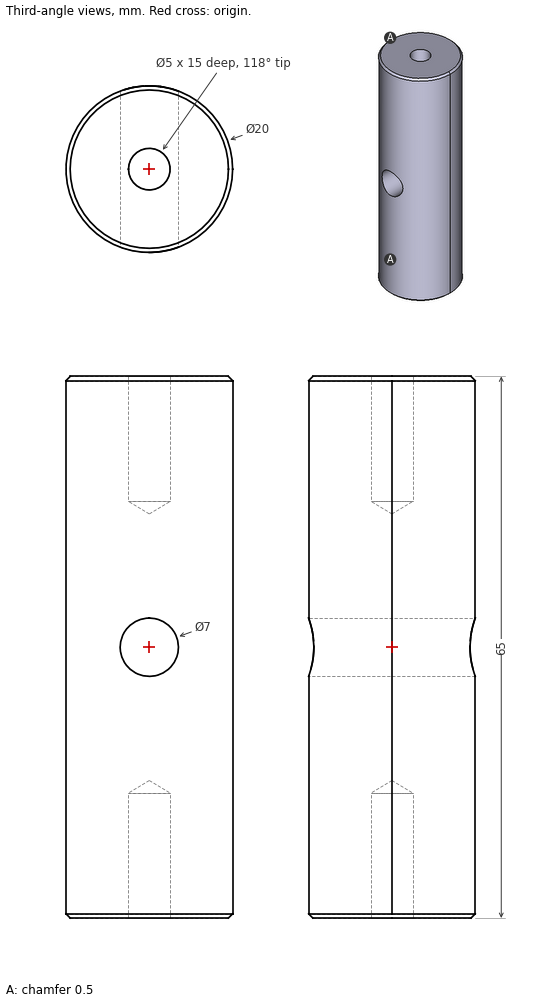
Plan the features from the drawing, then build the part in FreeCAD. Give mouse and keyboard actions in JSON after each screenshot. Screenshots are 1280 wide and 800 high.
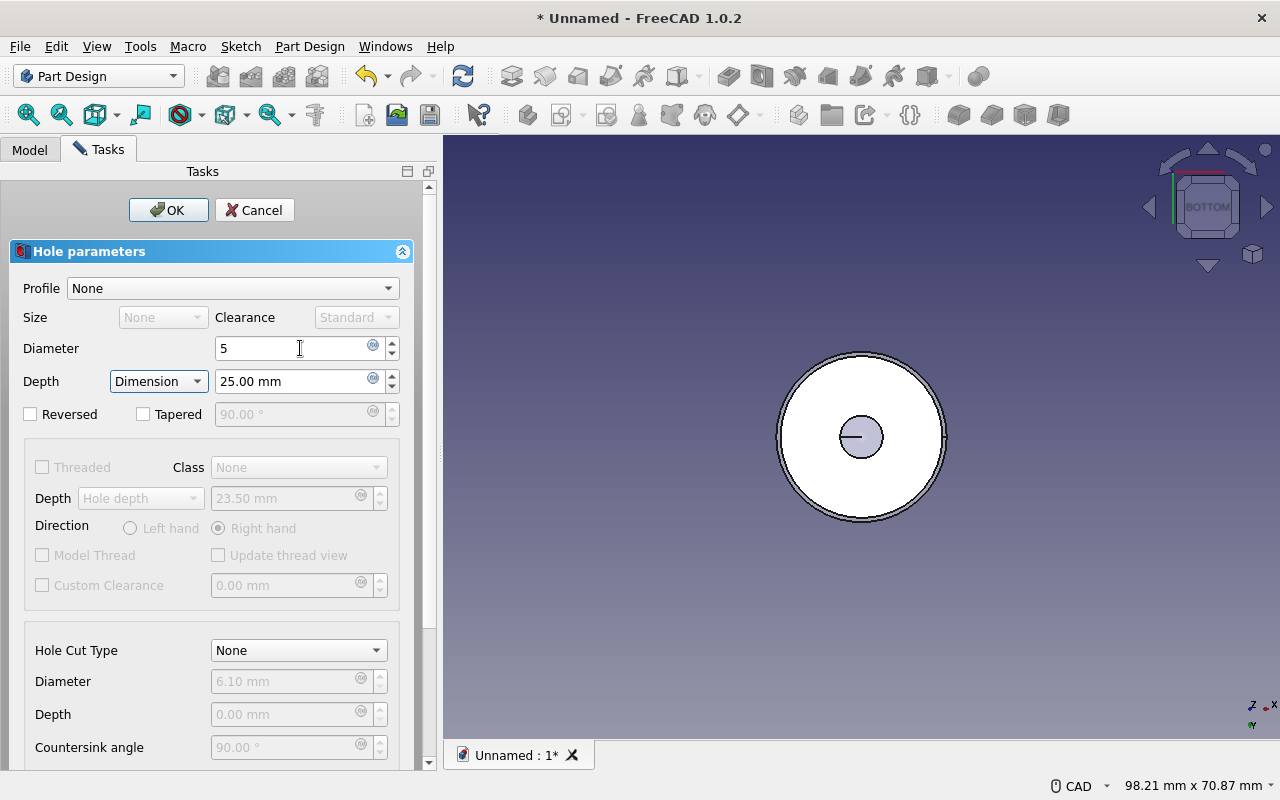
{"action": "triple_click", "coordinate": [300, 382]}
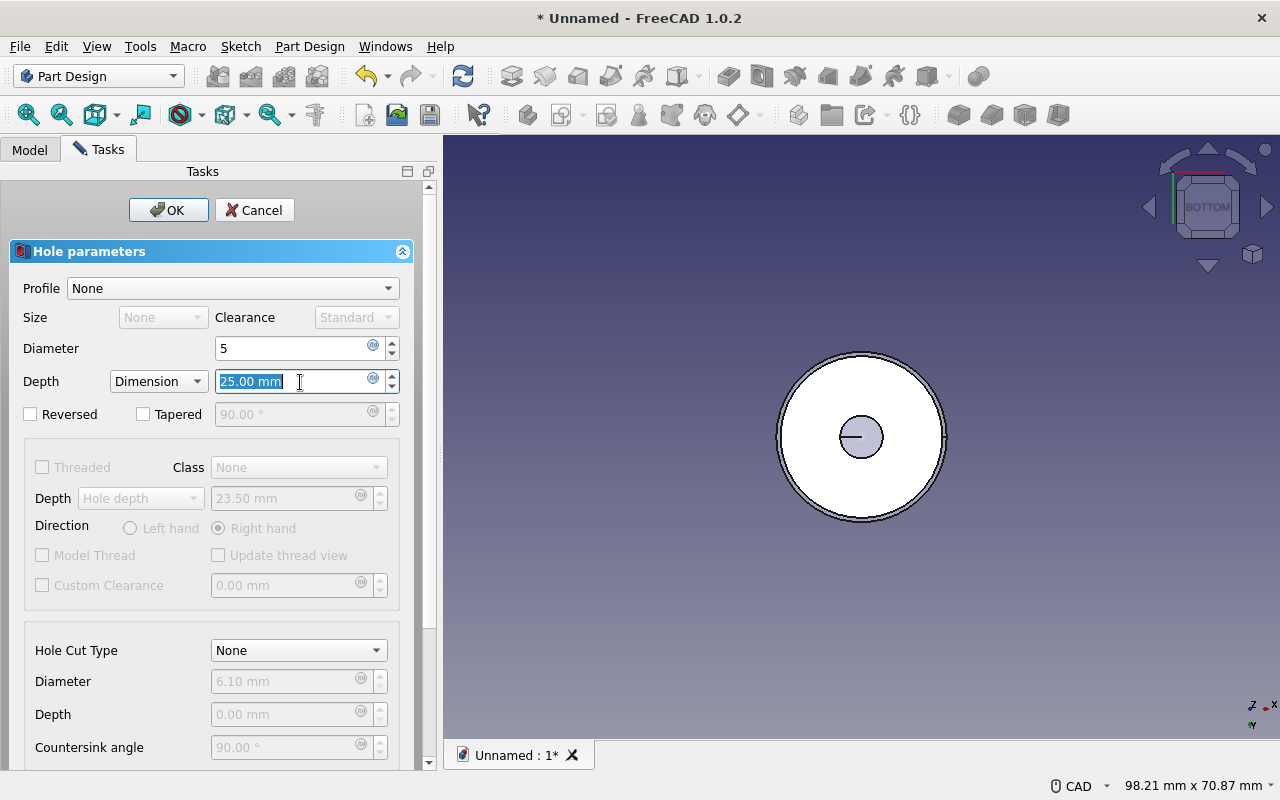
{"action": "type", "text": "15"}
{"action": "key", "text": "Tab"}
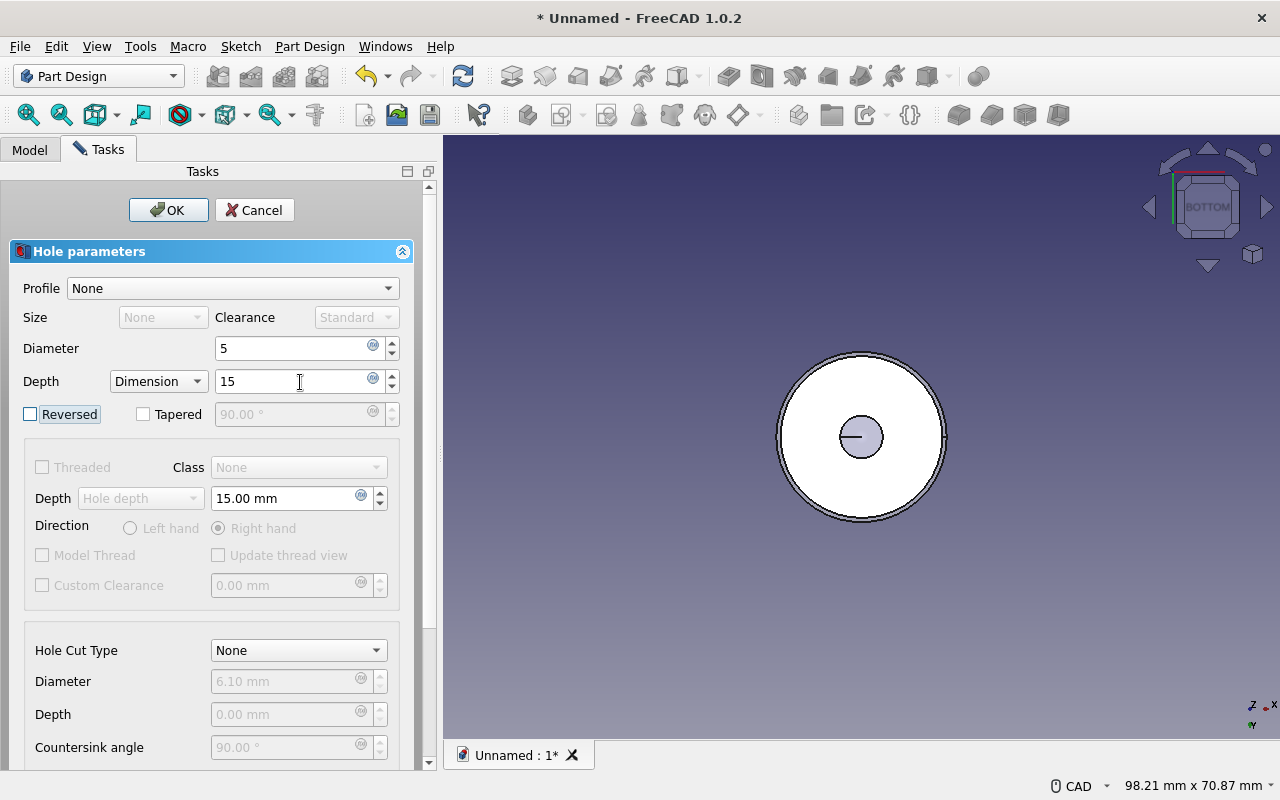
{"action": "left_click", "coordinate": [169, 210]}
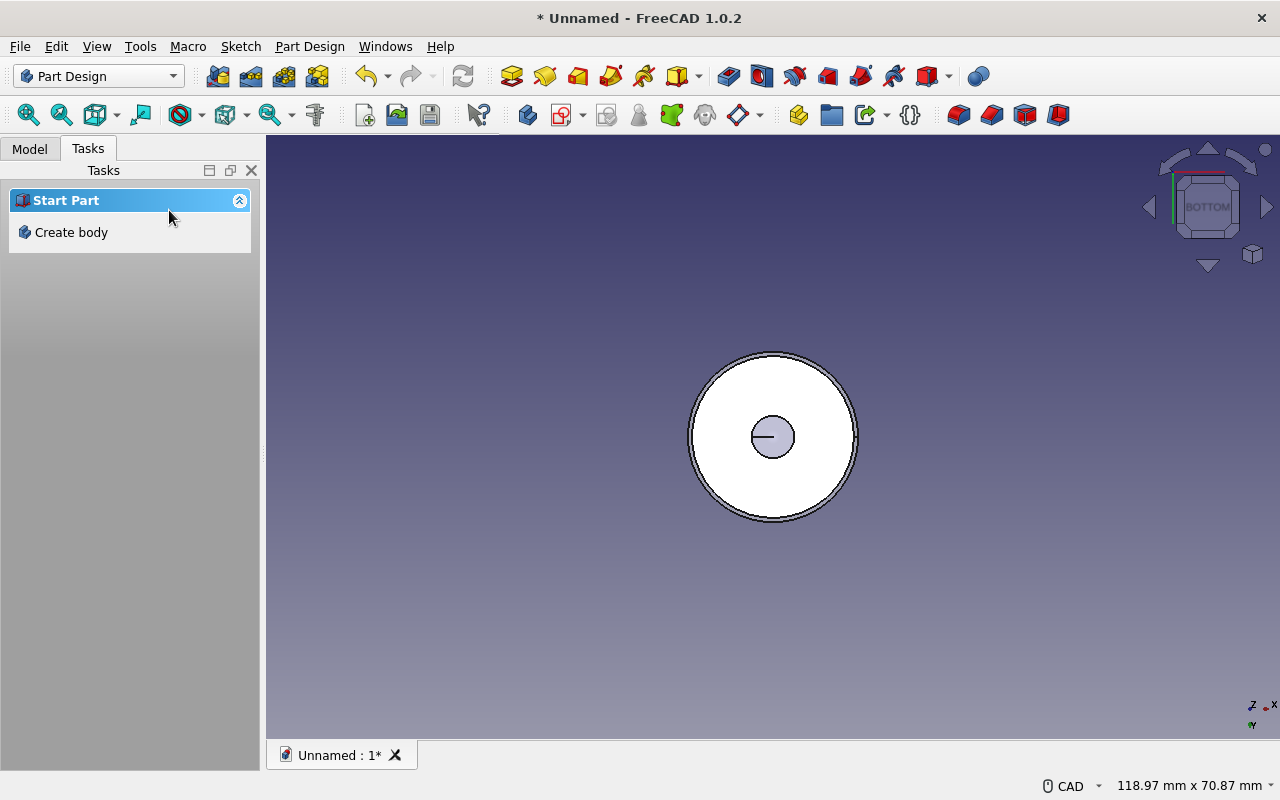
{"action": "left_click", "coordinate": [29, 116]}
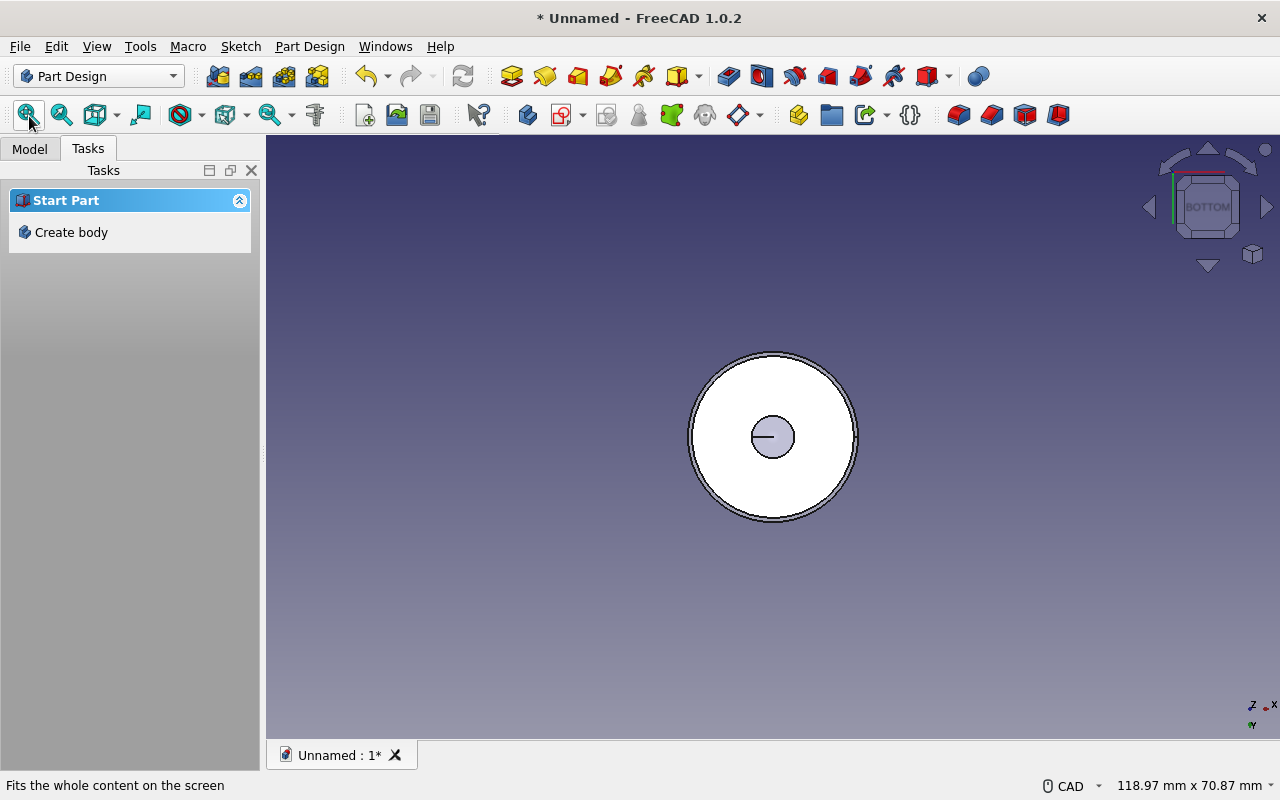
{"action": "left_click", "coordinate": [560, 116]}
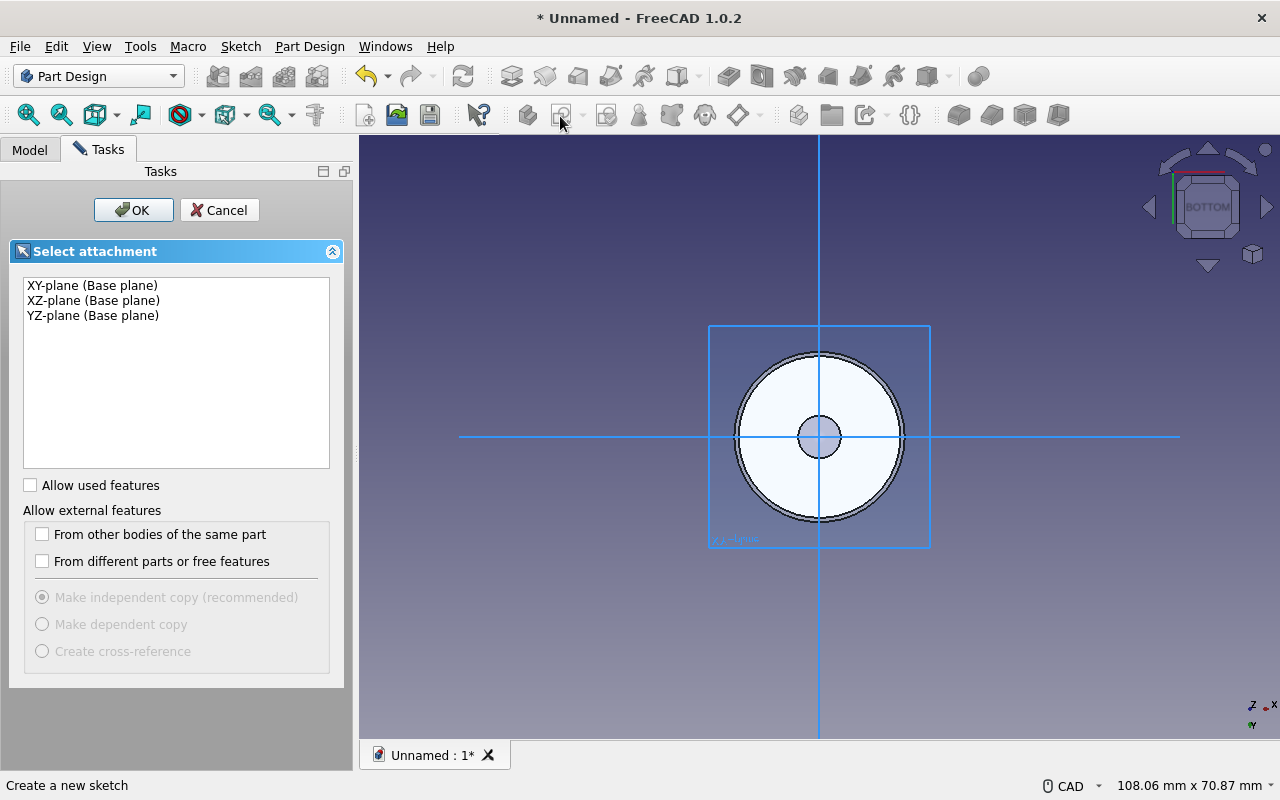
{"action": "left_click", "coordinate": [84, 300]}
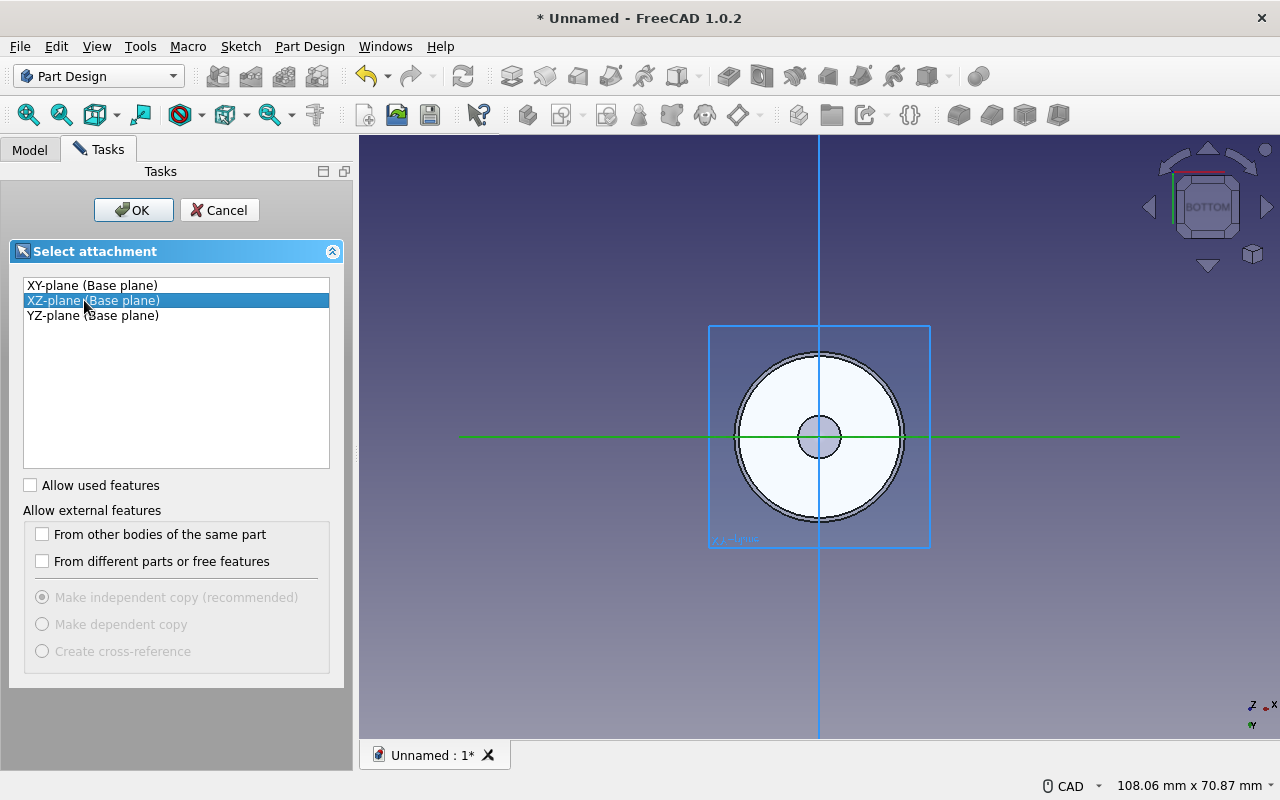
{"action": "left_click", "coordinate": [134, 210]}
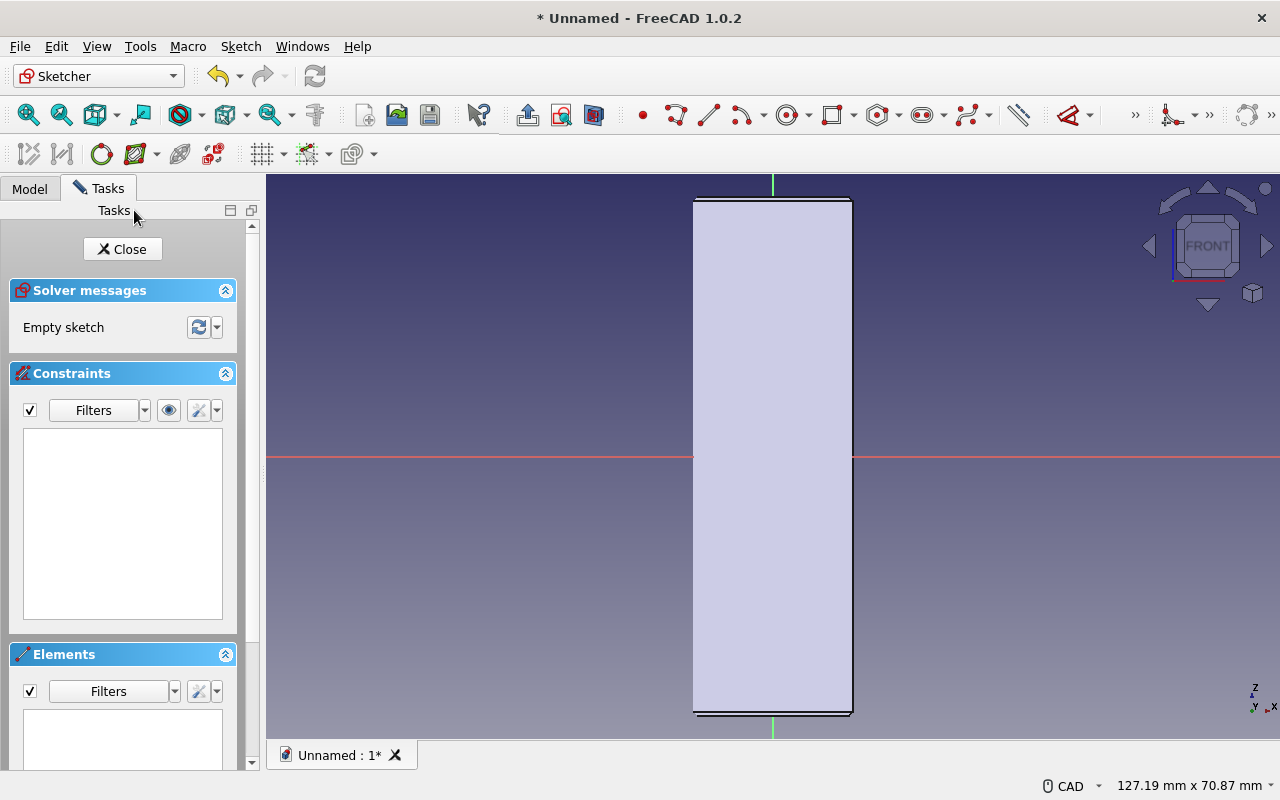
{"action": "left_click", "coordinate": [594, 116]}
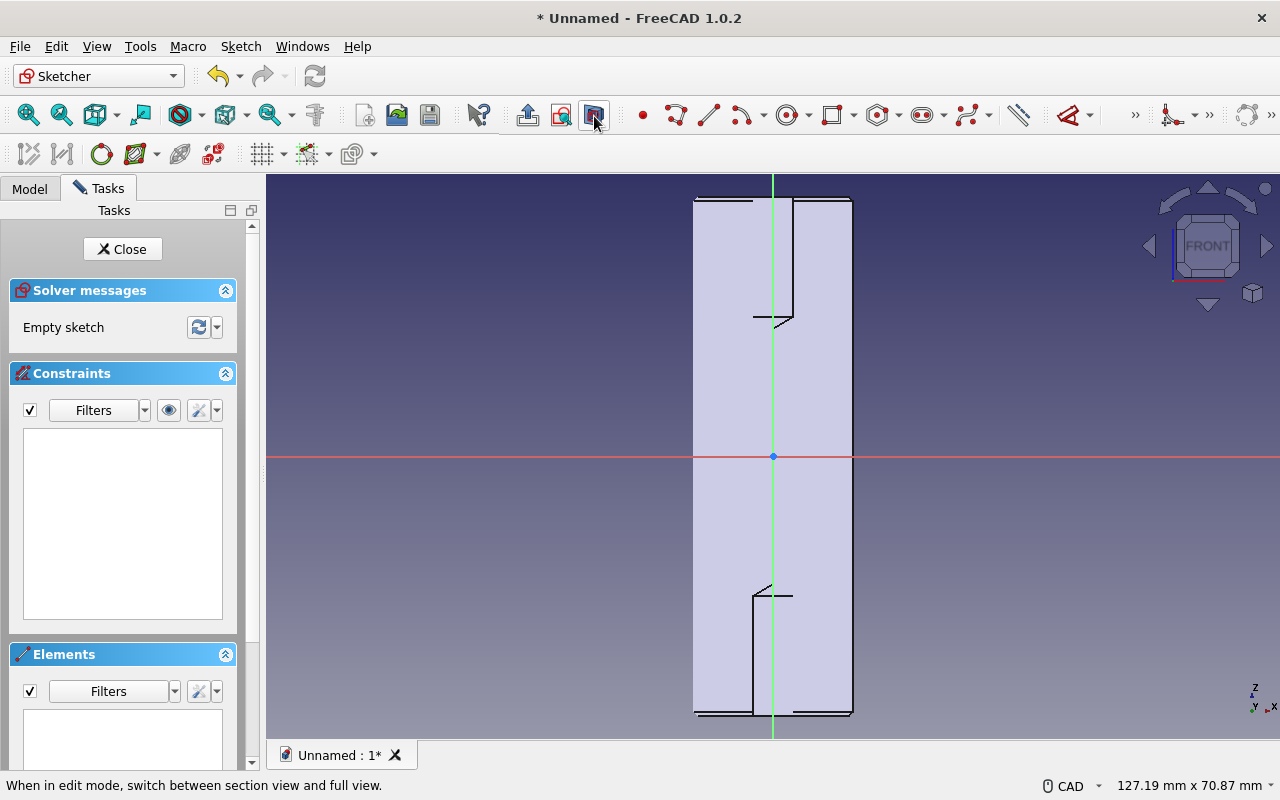
{"action": "scroll", "coordinate": [787, 456], "scroll_direction": "up", "scroll_amount": 9}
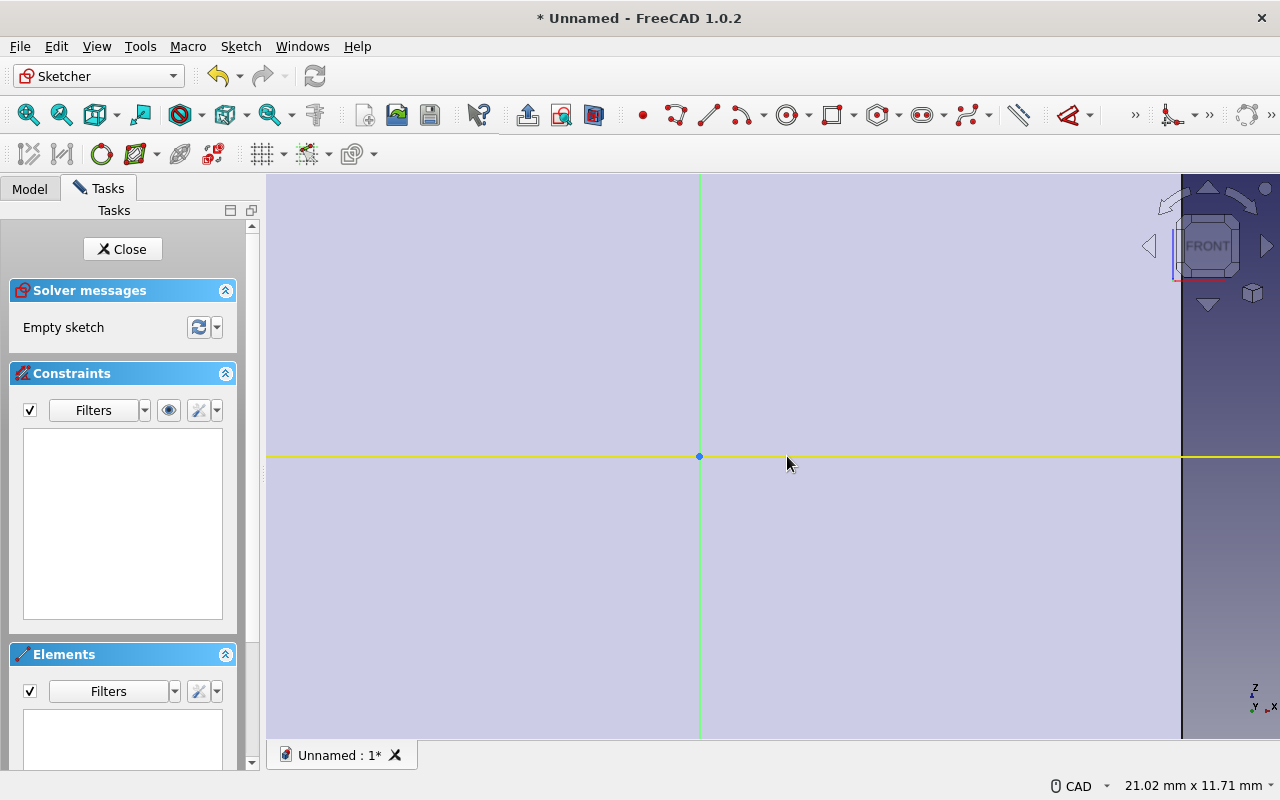
{"action": "left_click", "coordinate": [786, 116]}